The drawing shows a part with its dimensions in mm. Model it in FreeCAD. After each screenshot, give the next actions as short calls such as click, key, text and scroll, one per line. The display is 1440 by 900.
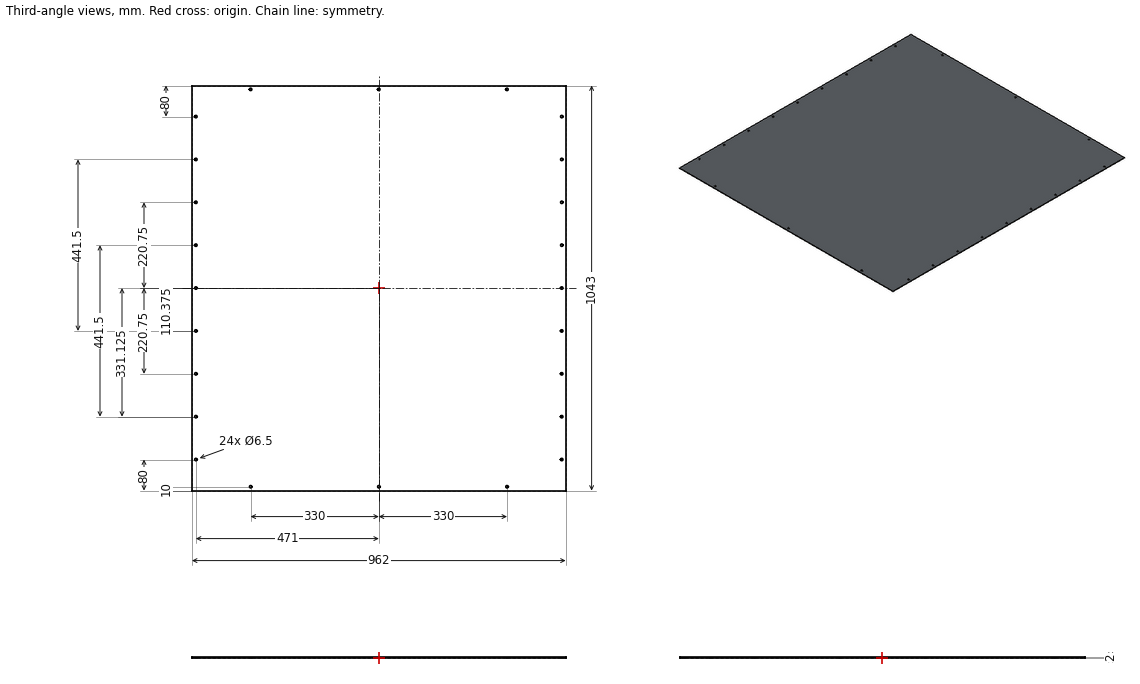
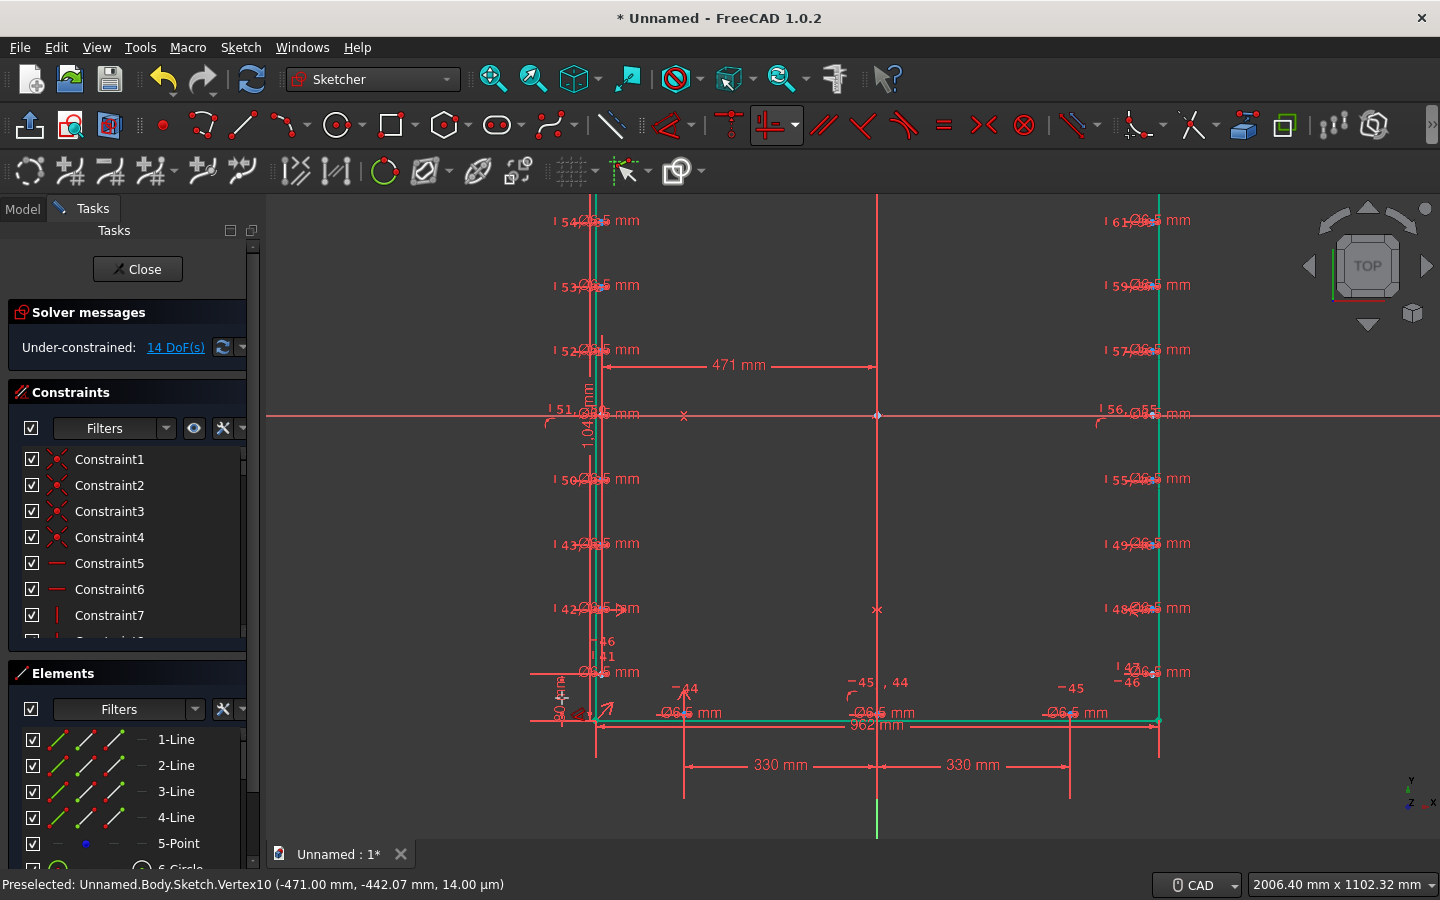
scroll(596, 721, up, 10)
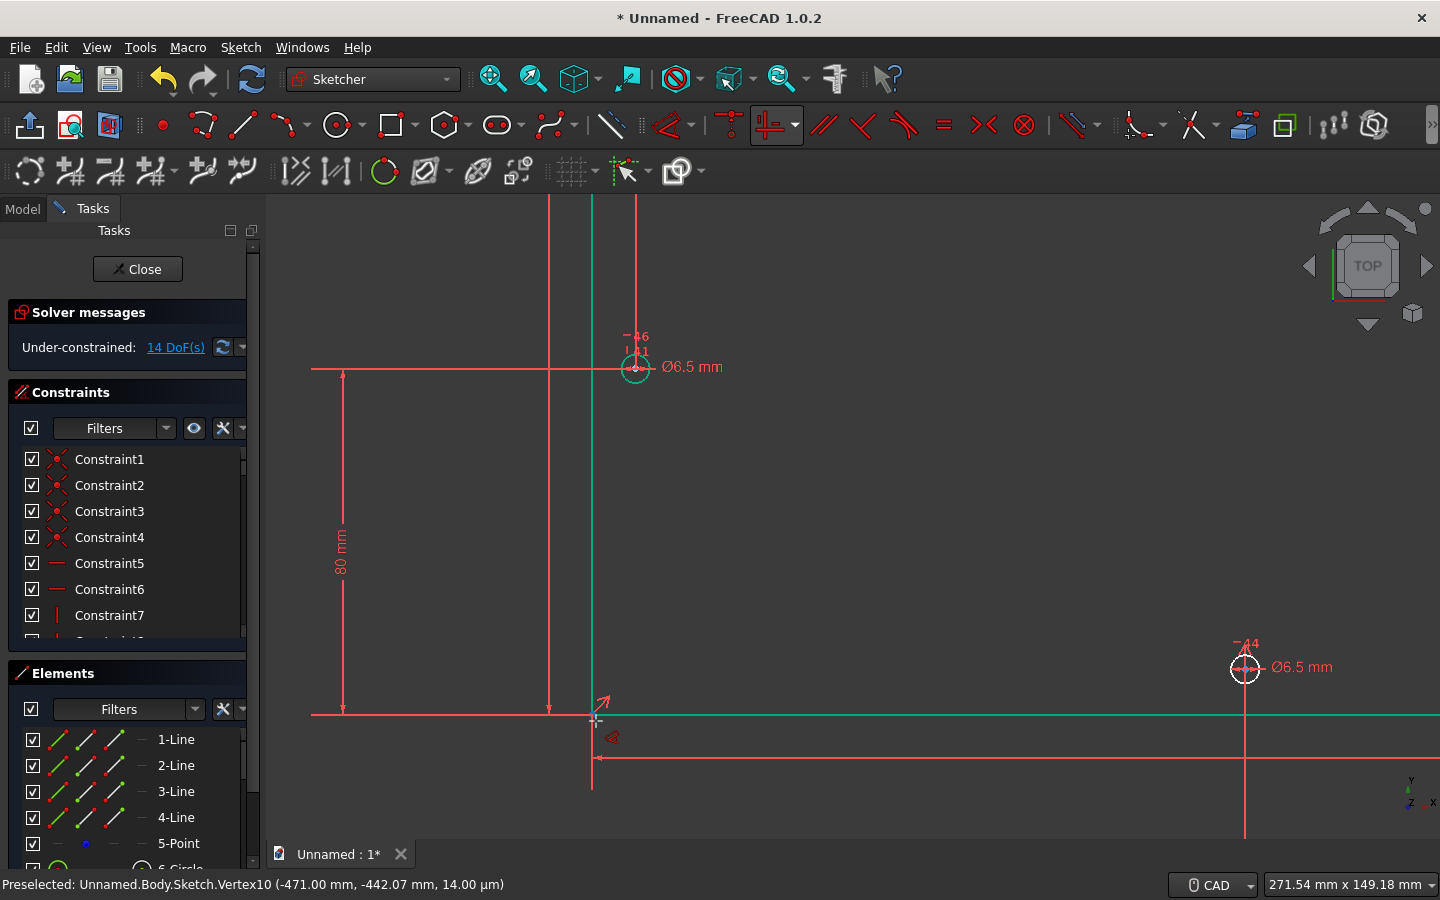
click(592, 715)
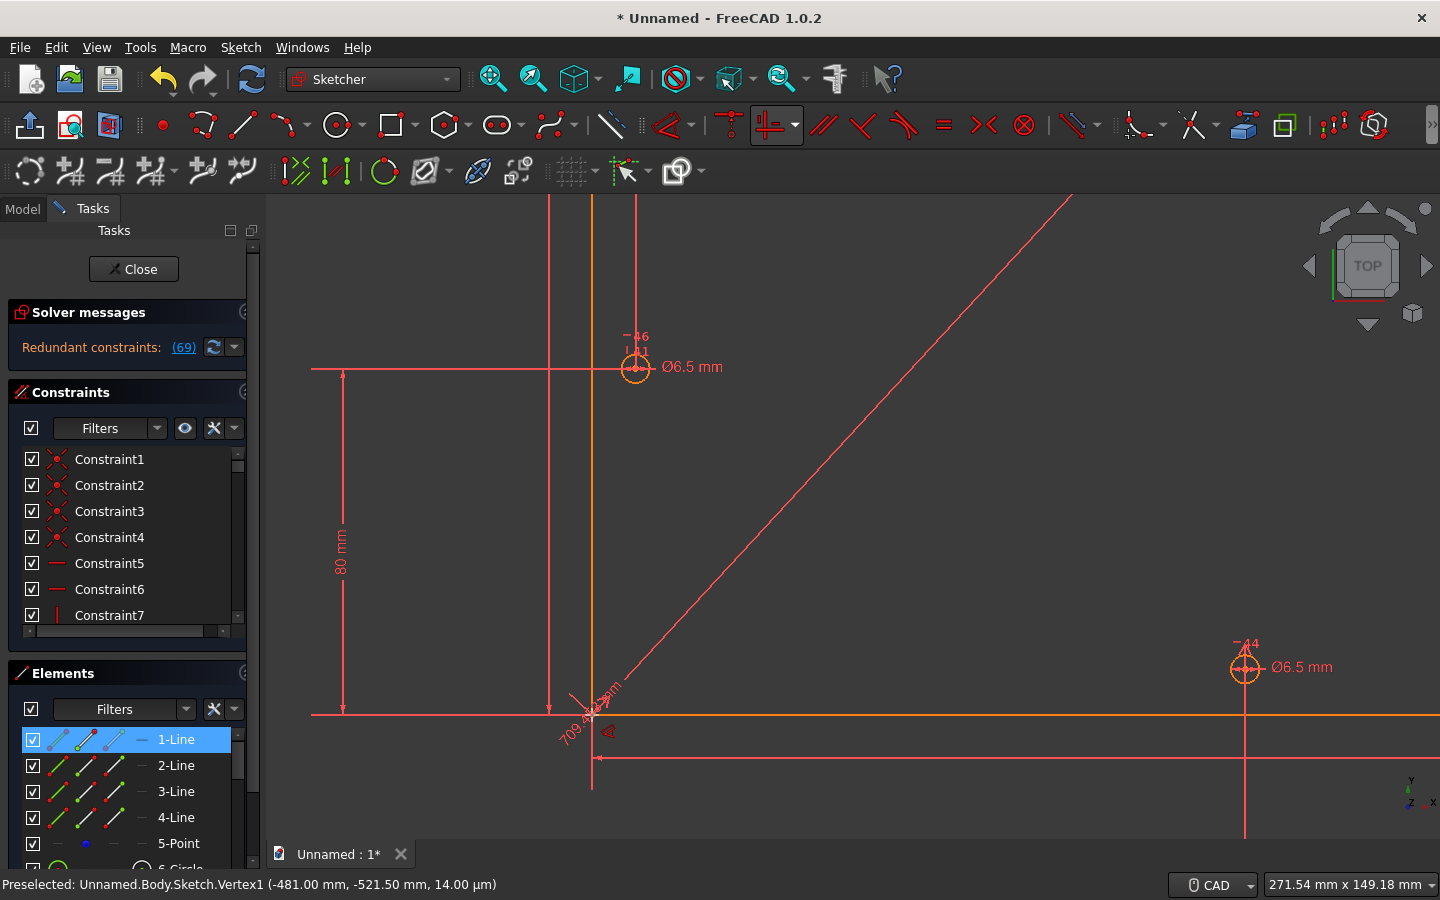
click(1245, 669)
click(558, 692)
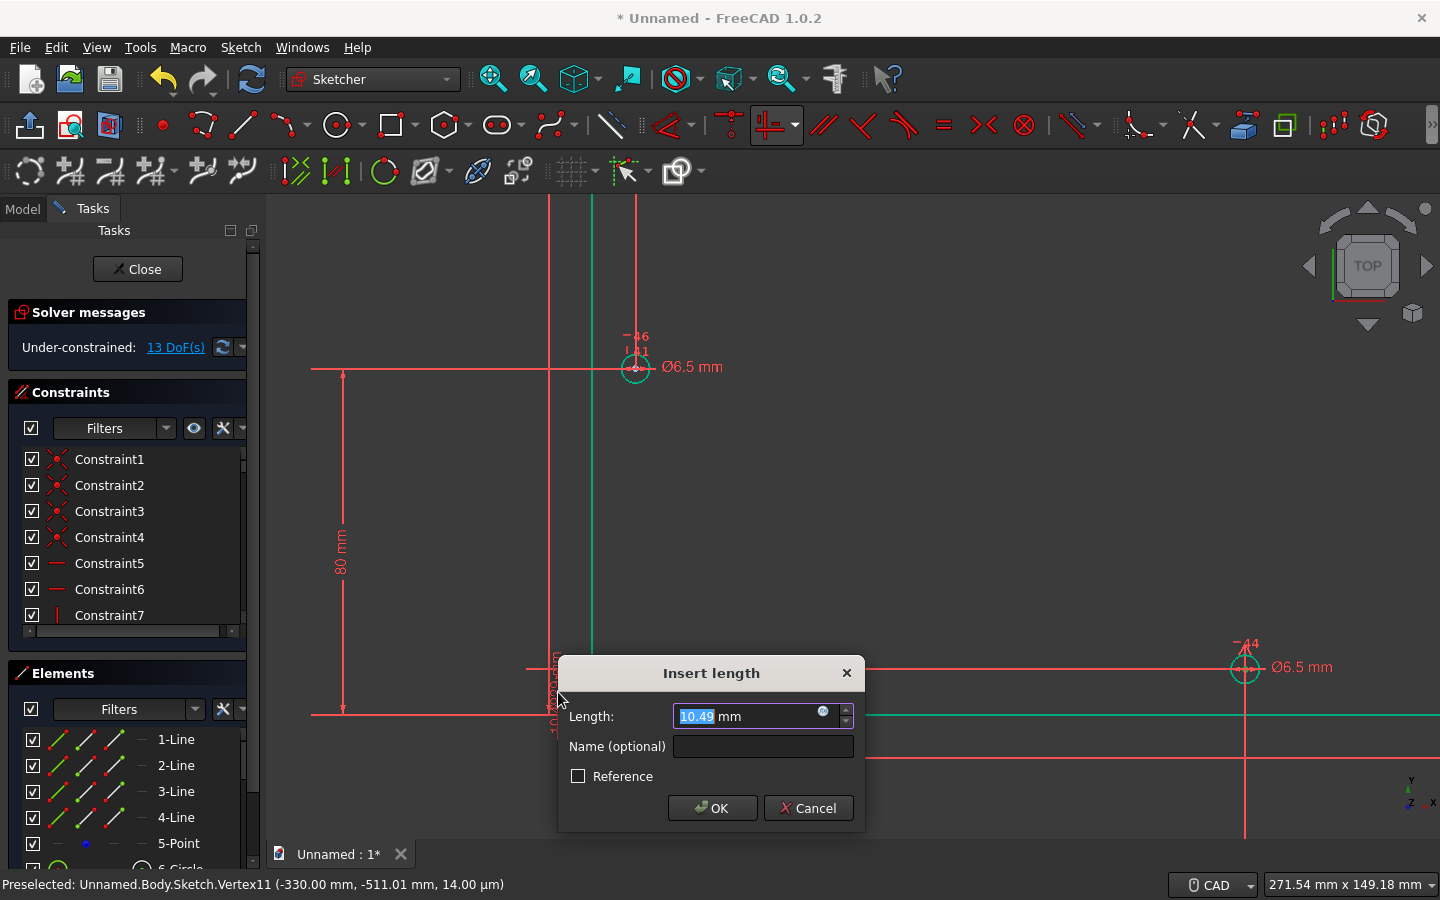
text(10)
key(Return)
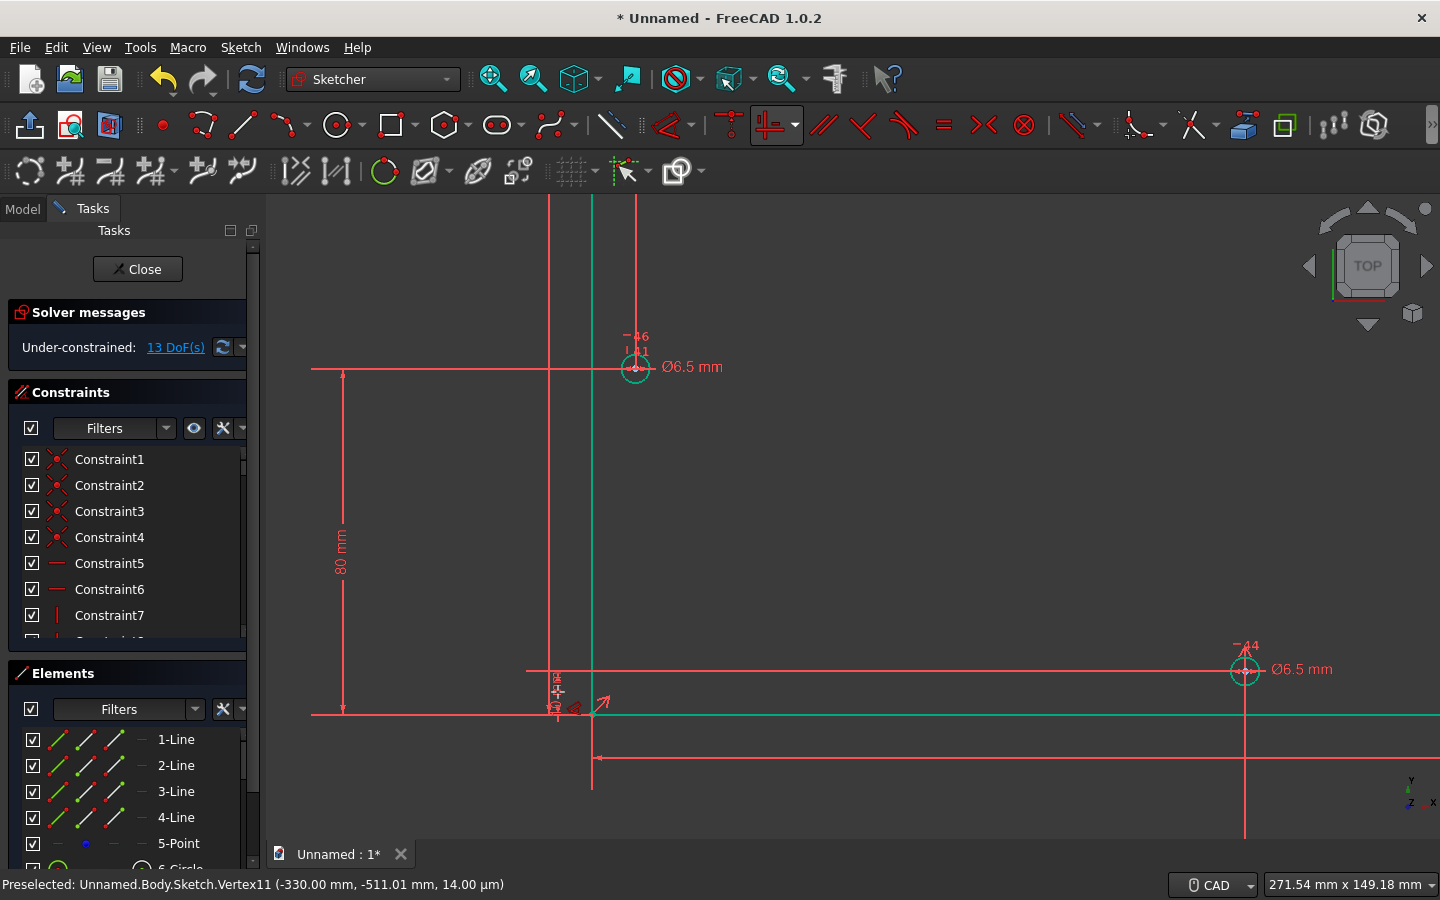
scroll(596, 722, down, 12)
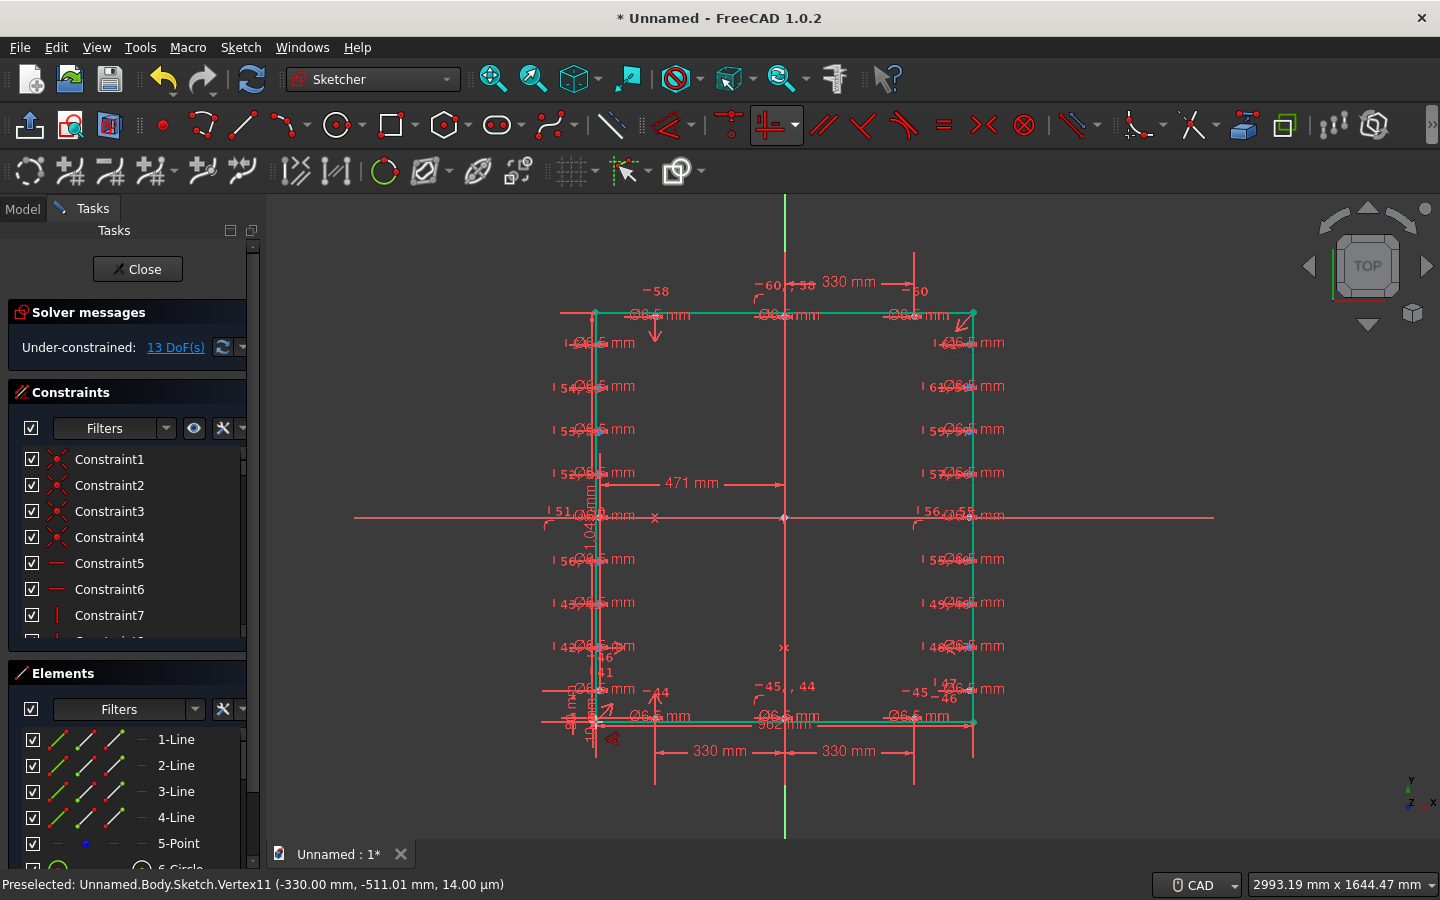
scroll(596, 313, up, 2)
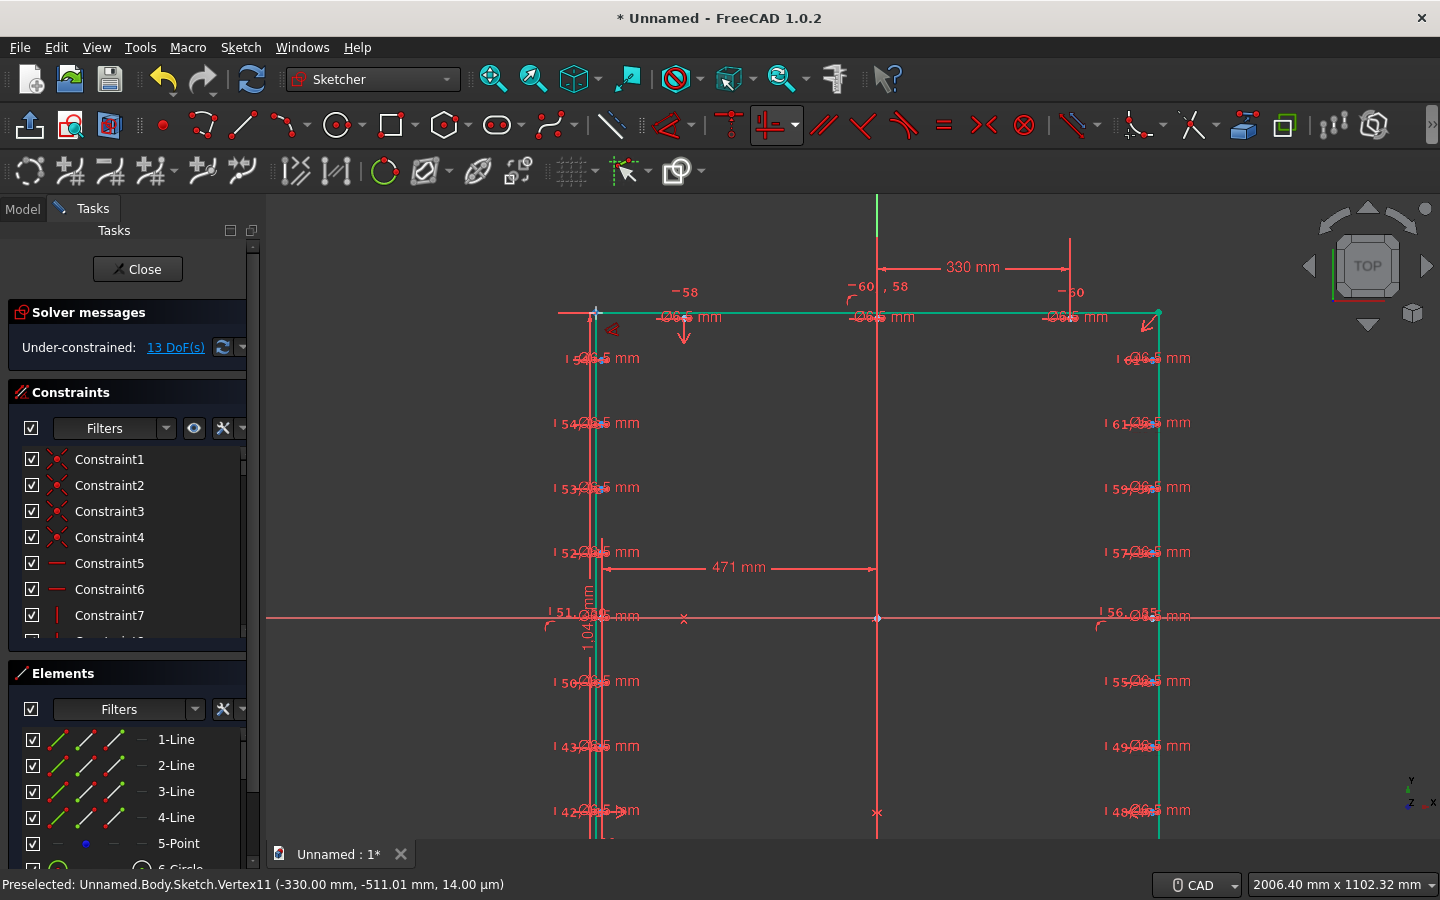
click(596, 313)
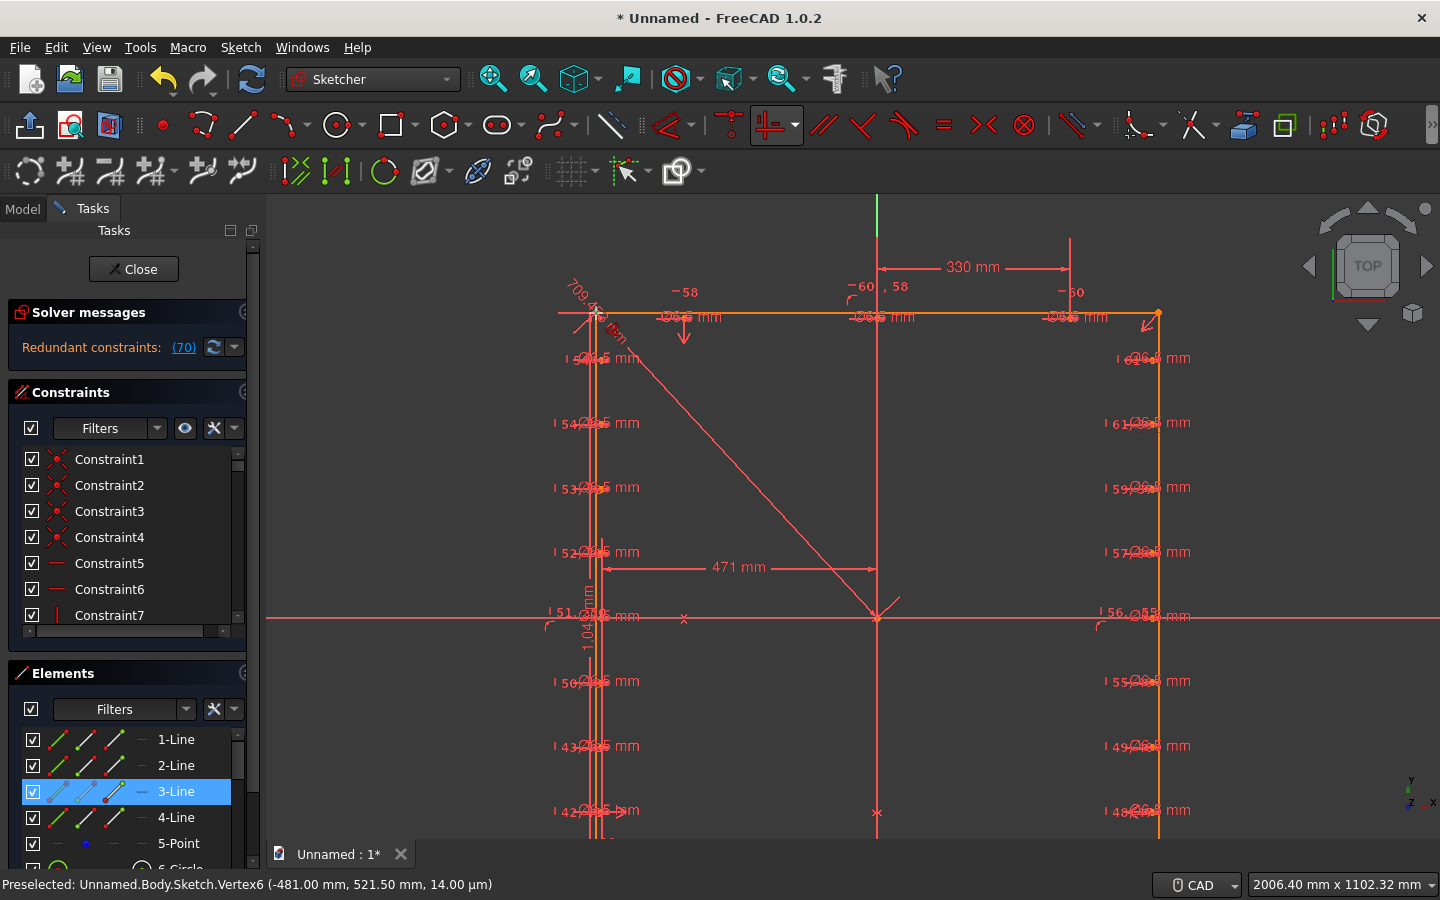
click(602, 360)
click(562, 337)